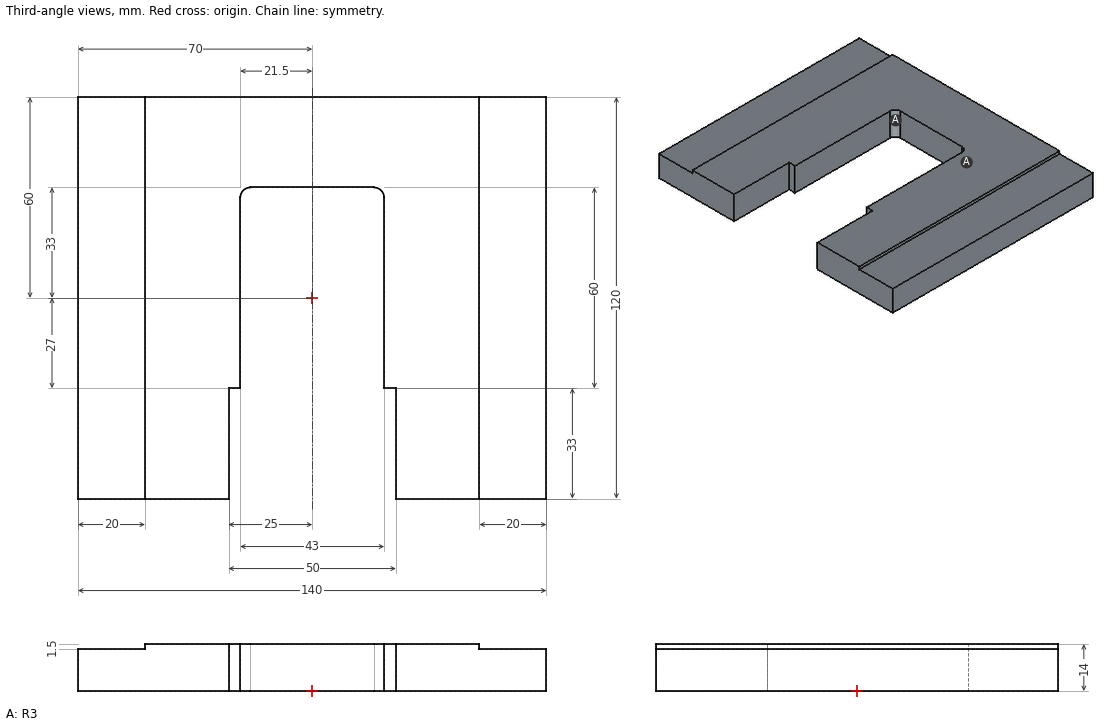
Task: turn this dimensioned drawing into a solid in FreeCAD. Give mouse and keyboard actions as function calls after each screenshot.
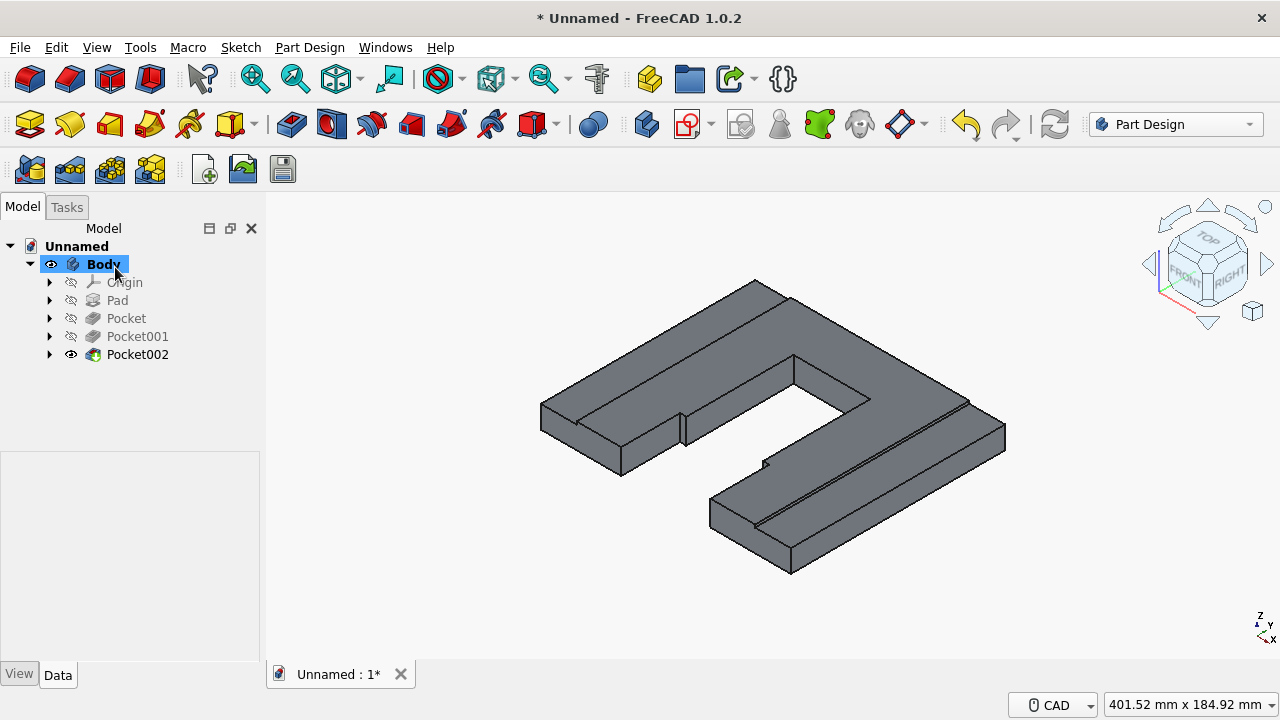
key(2)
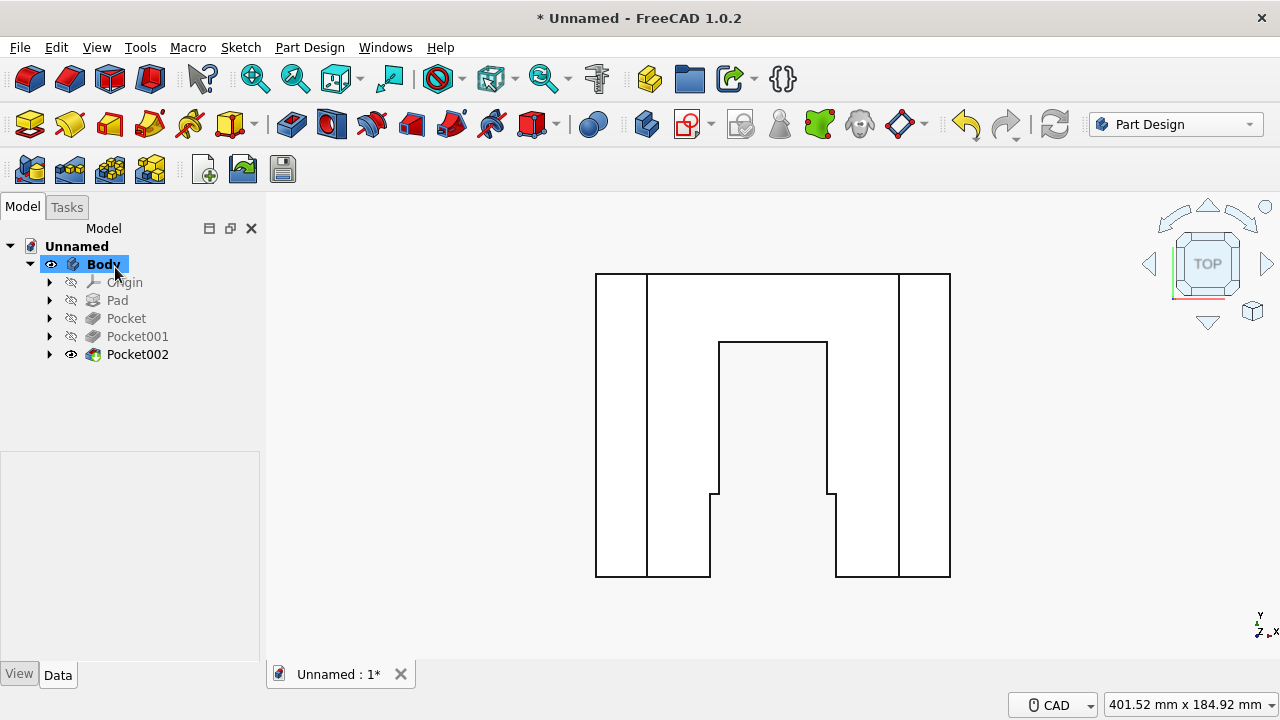
key(1)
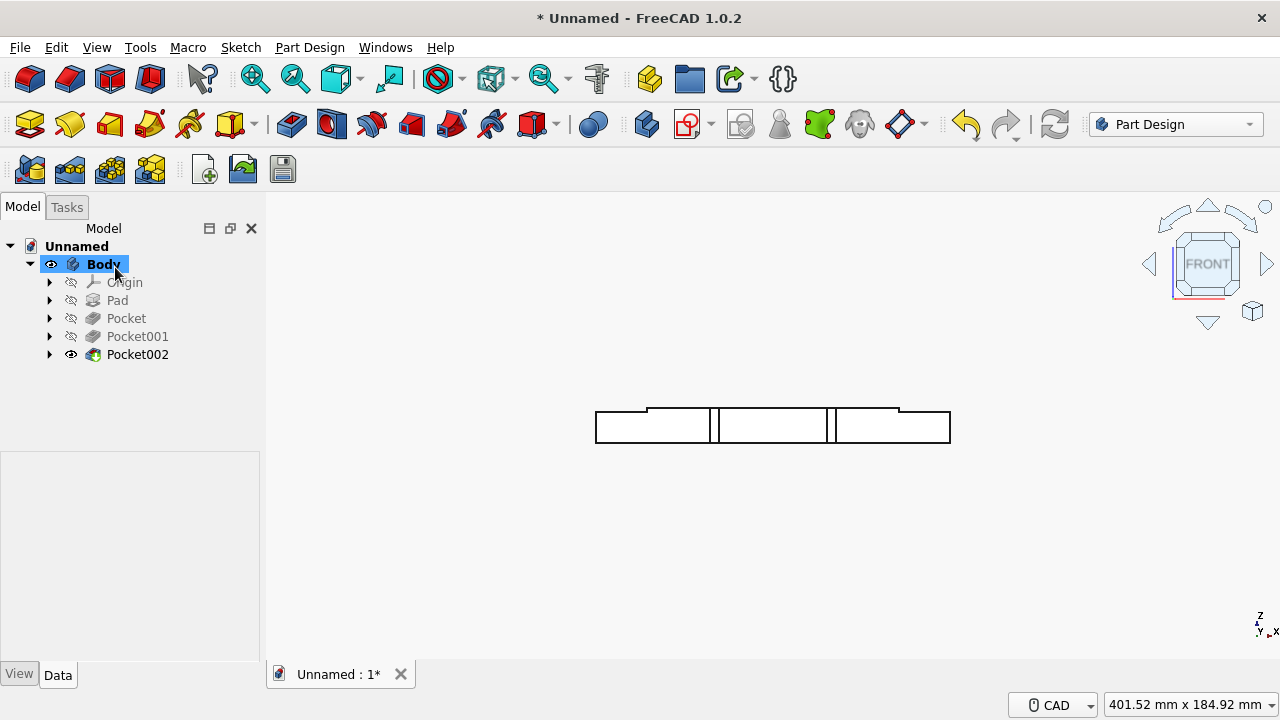
click(256, 80)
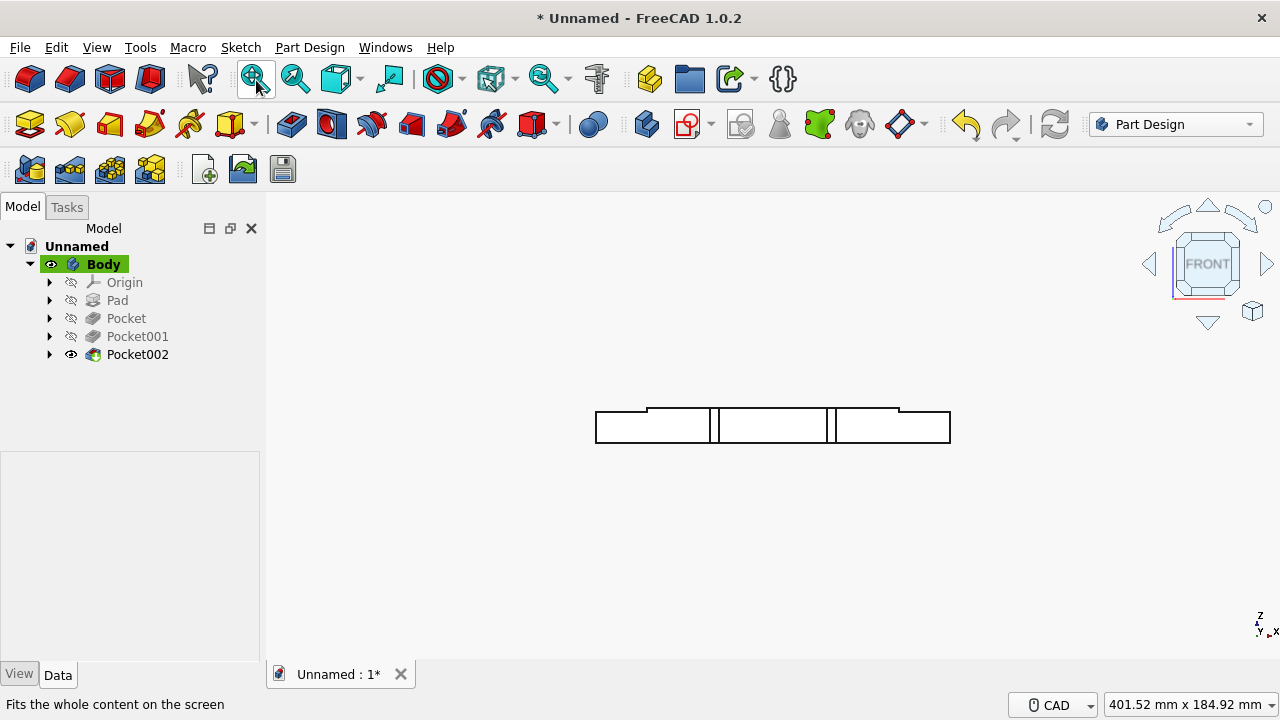
key(3)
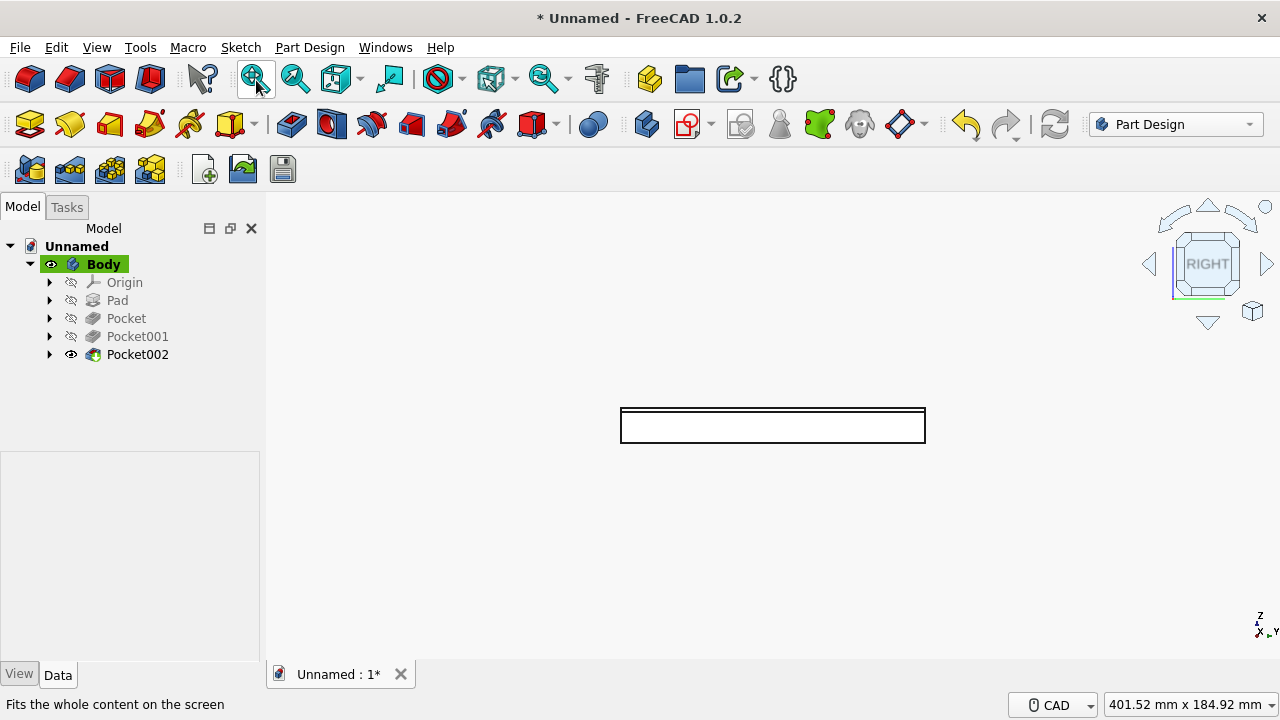
click(256, 80)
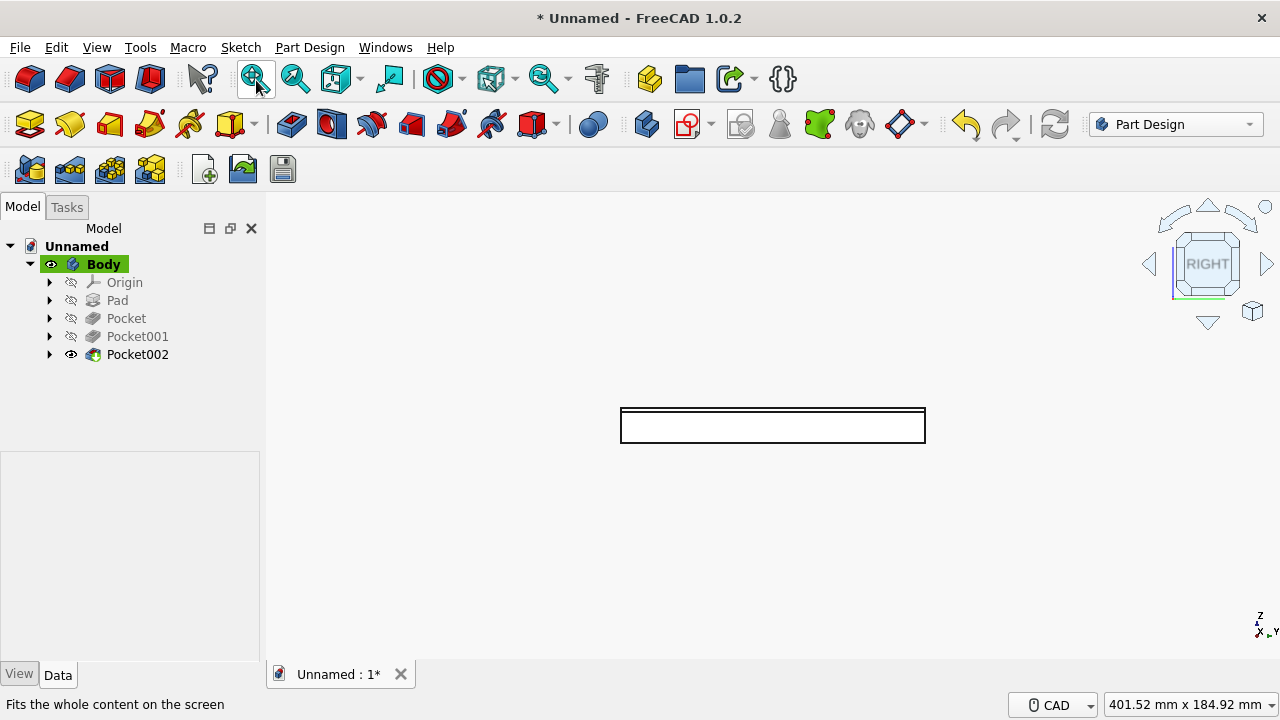
key(5)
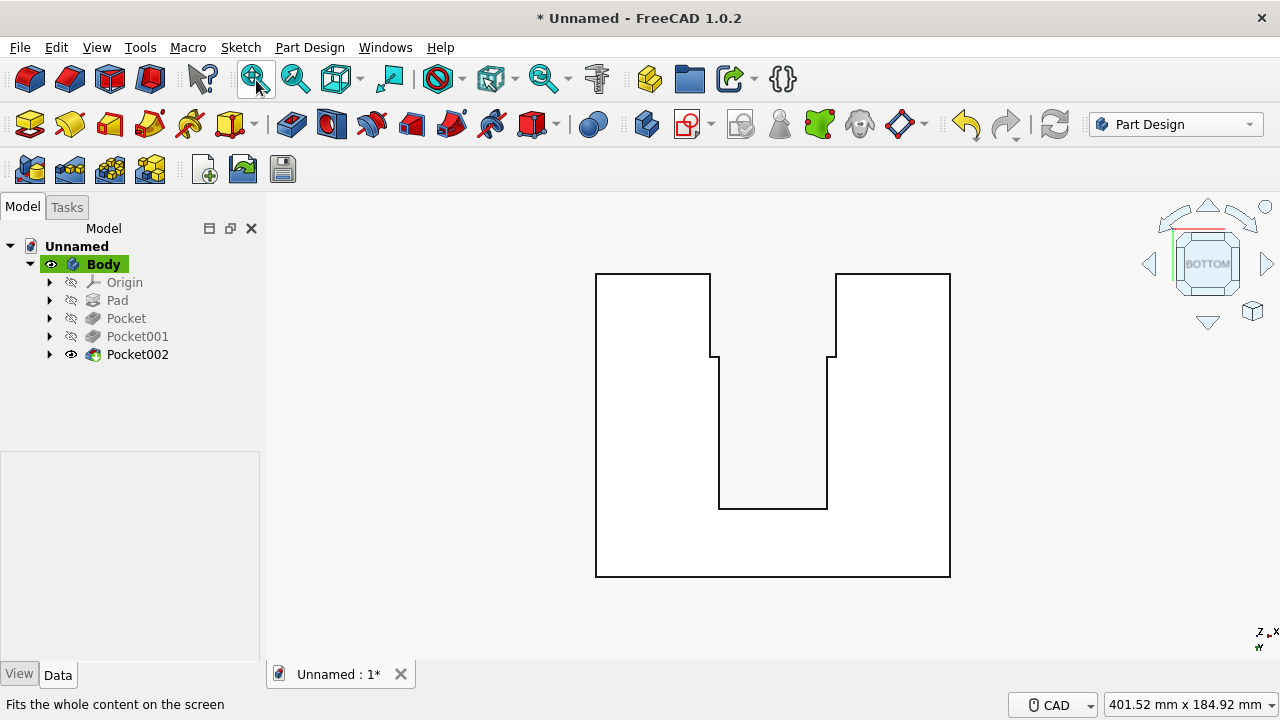
key(4)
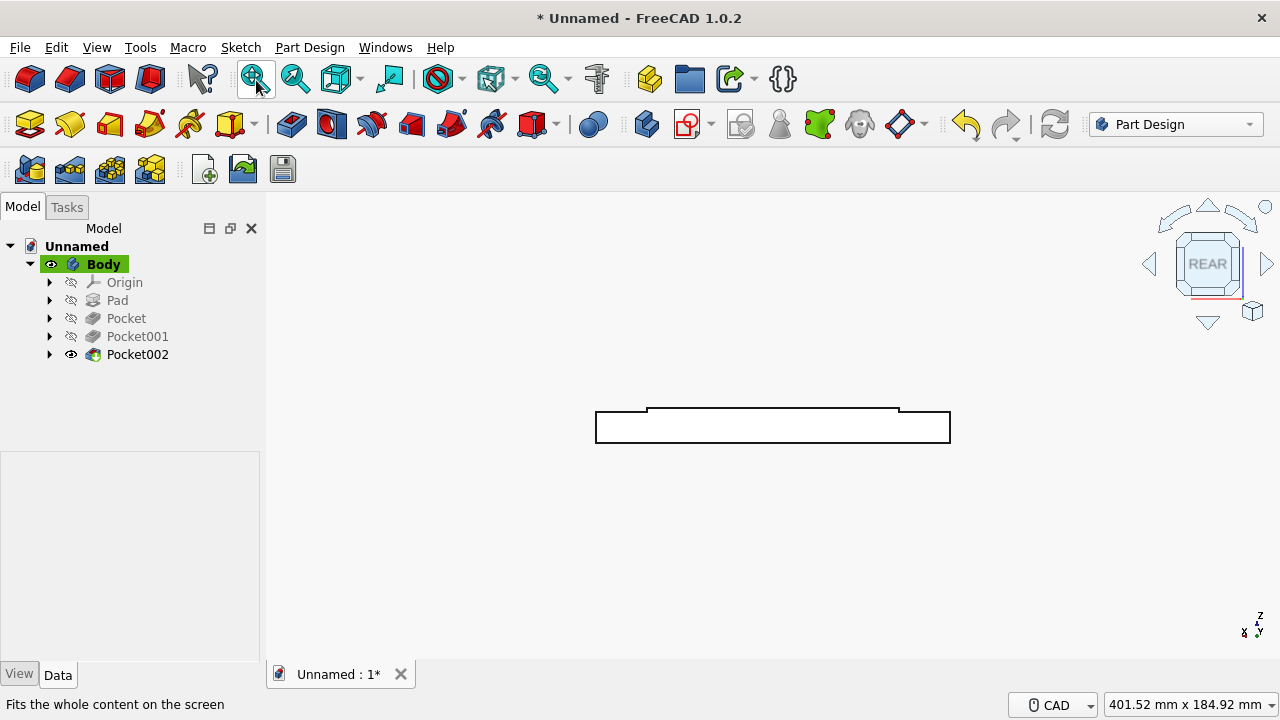
click(256, 80)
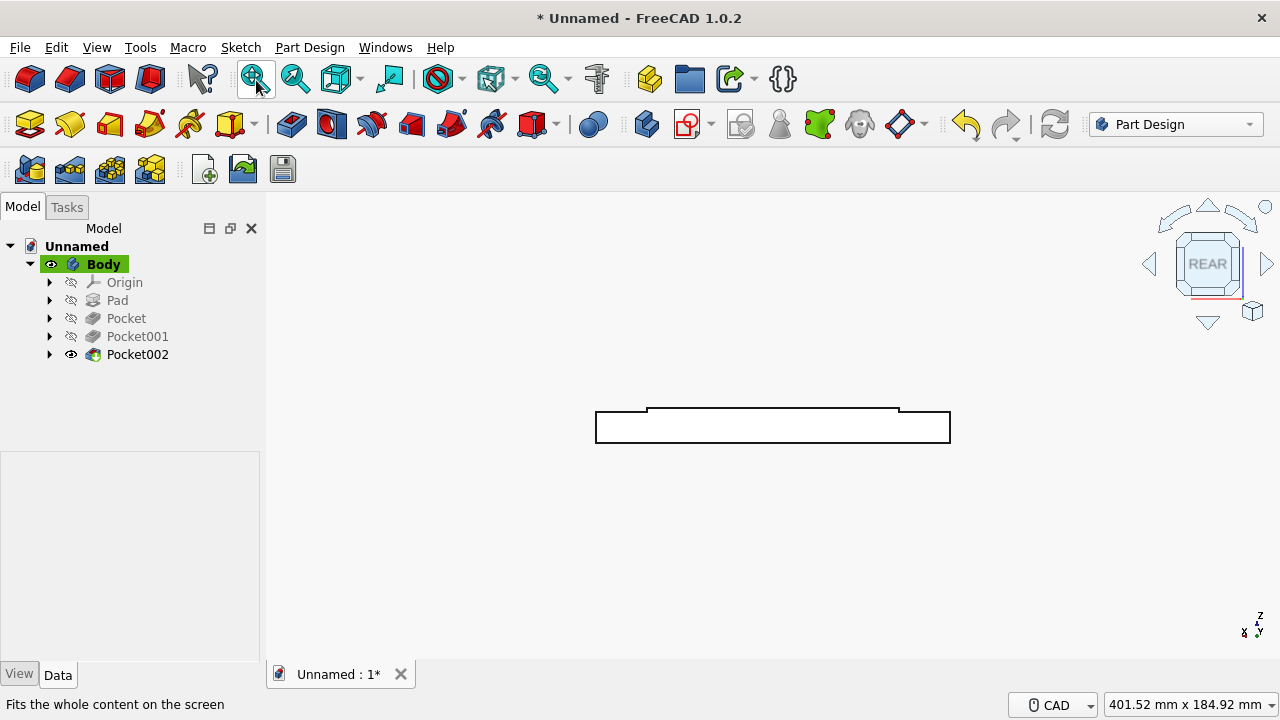
key(6)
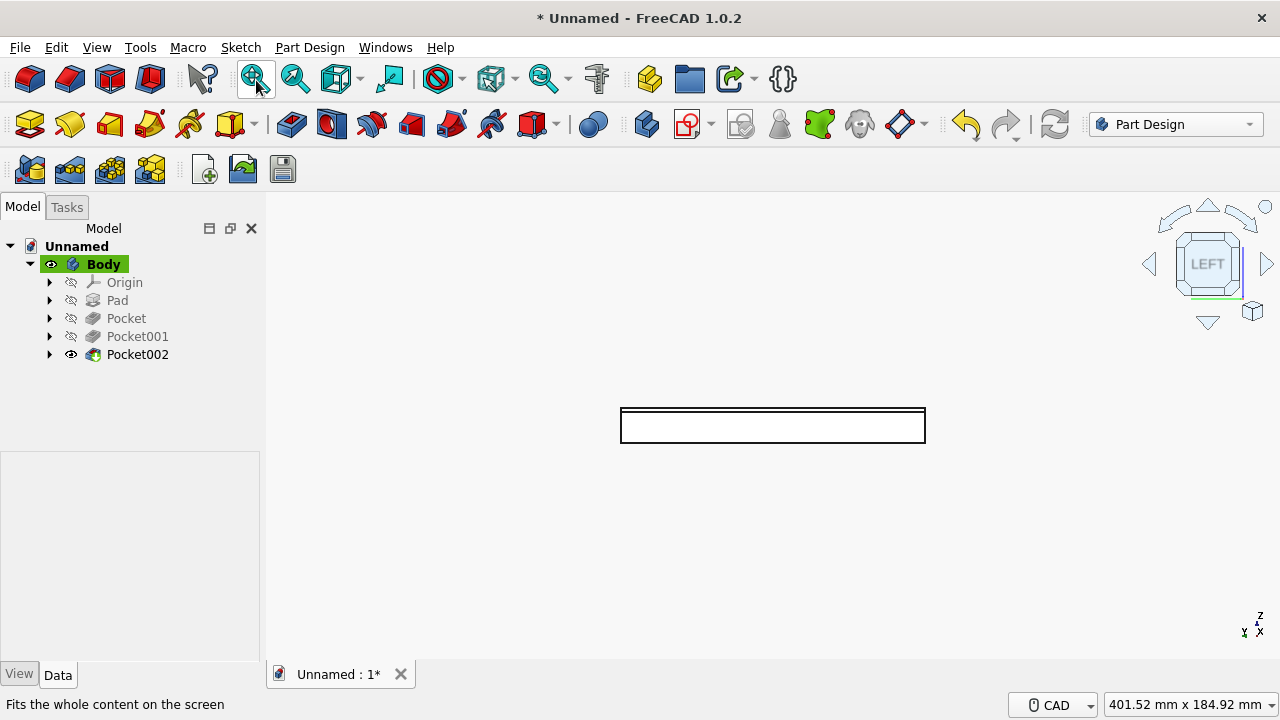
click(256, 80)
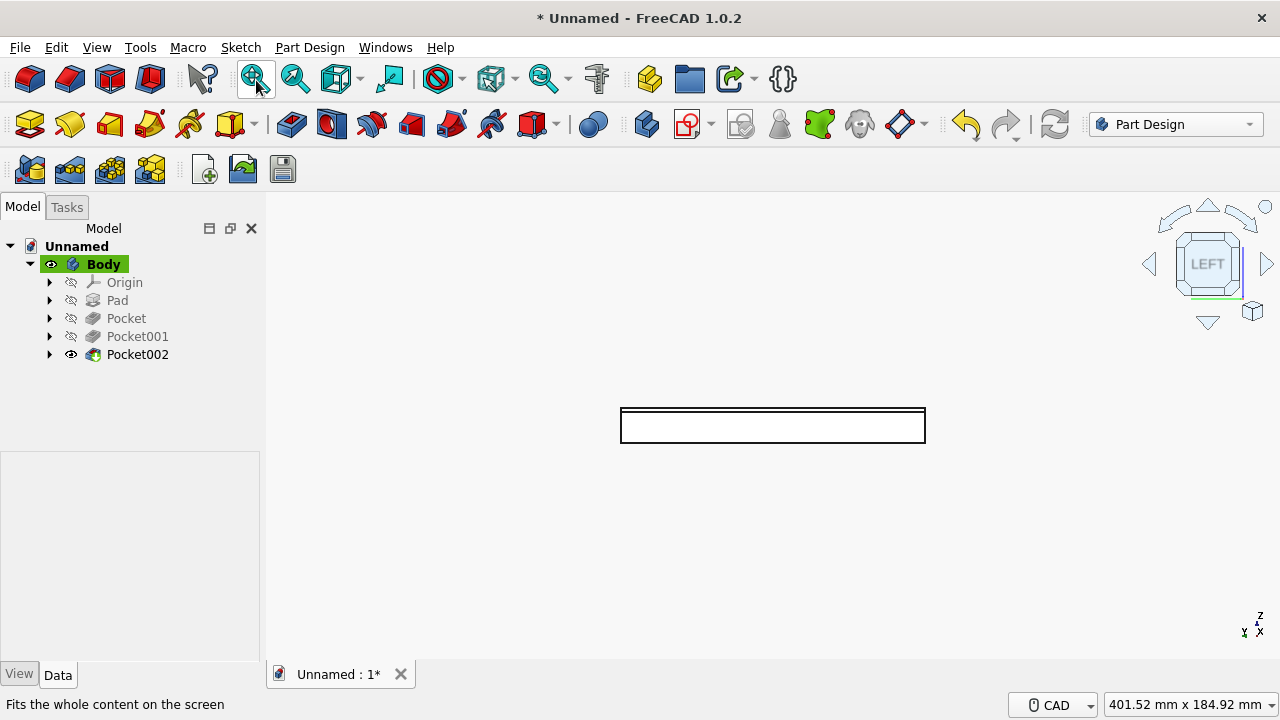
key(v)
key(3)